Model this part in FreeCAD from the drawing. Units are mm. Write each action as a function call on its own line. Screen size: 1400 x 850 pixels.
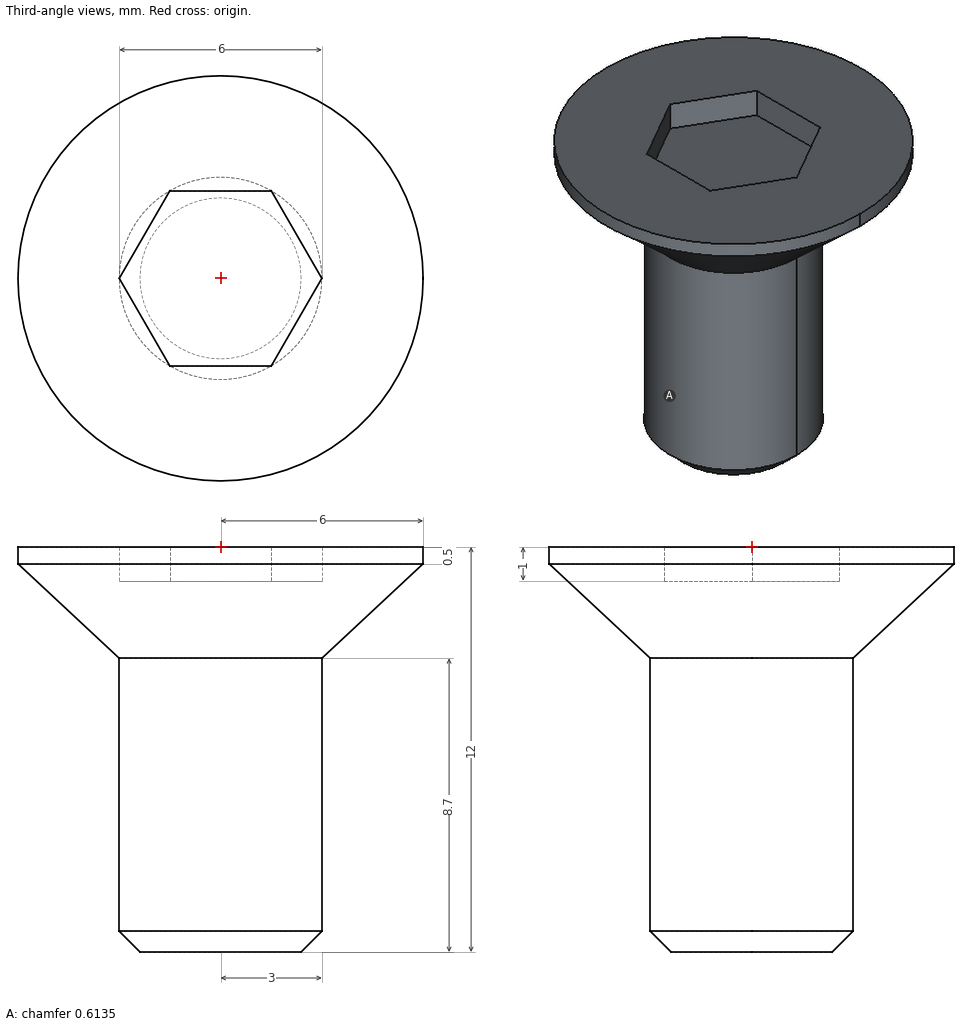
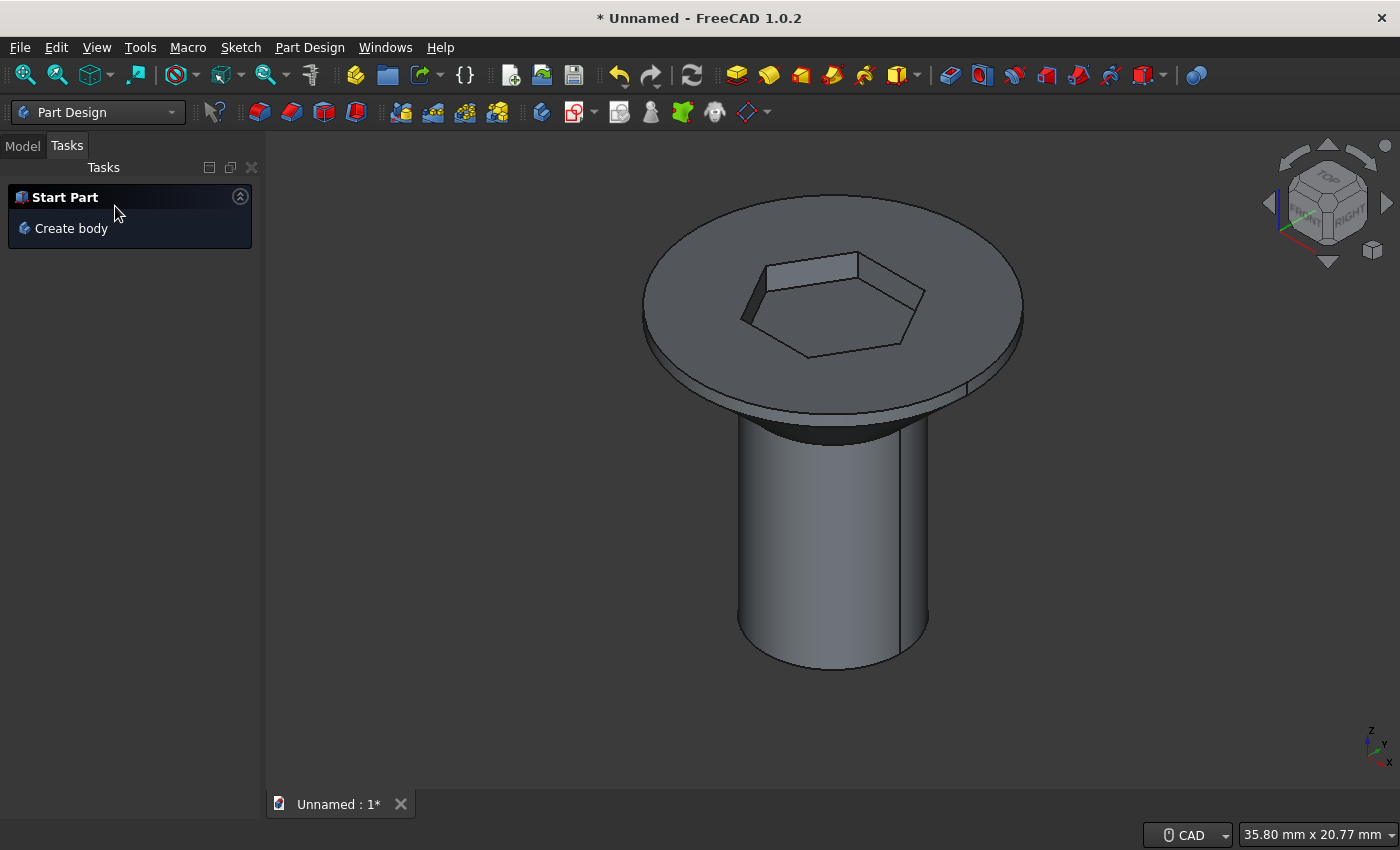
key(2)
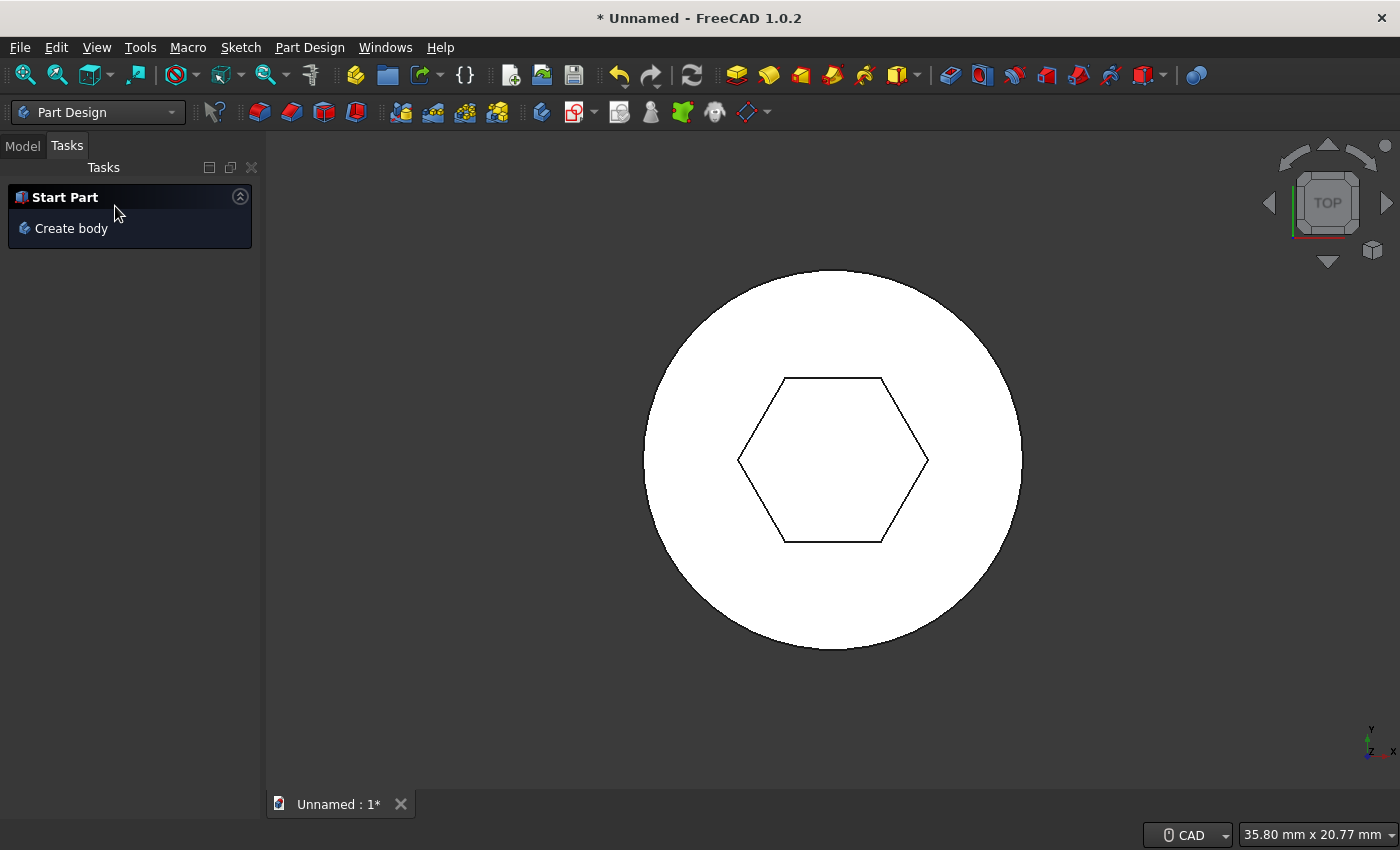
key(1)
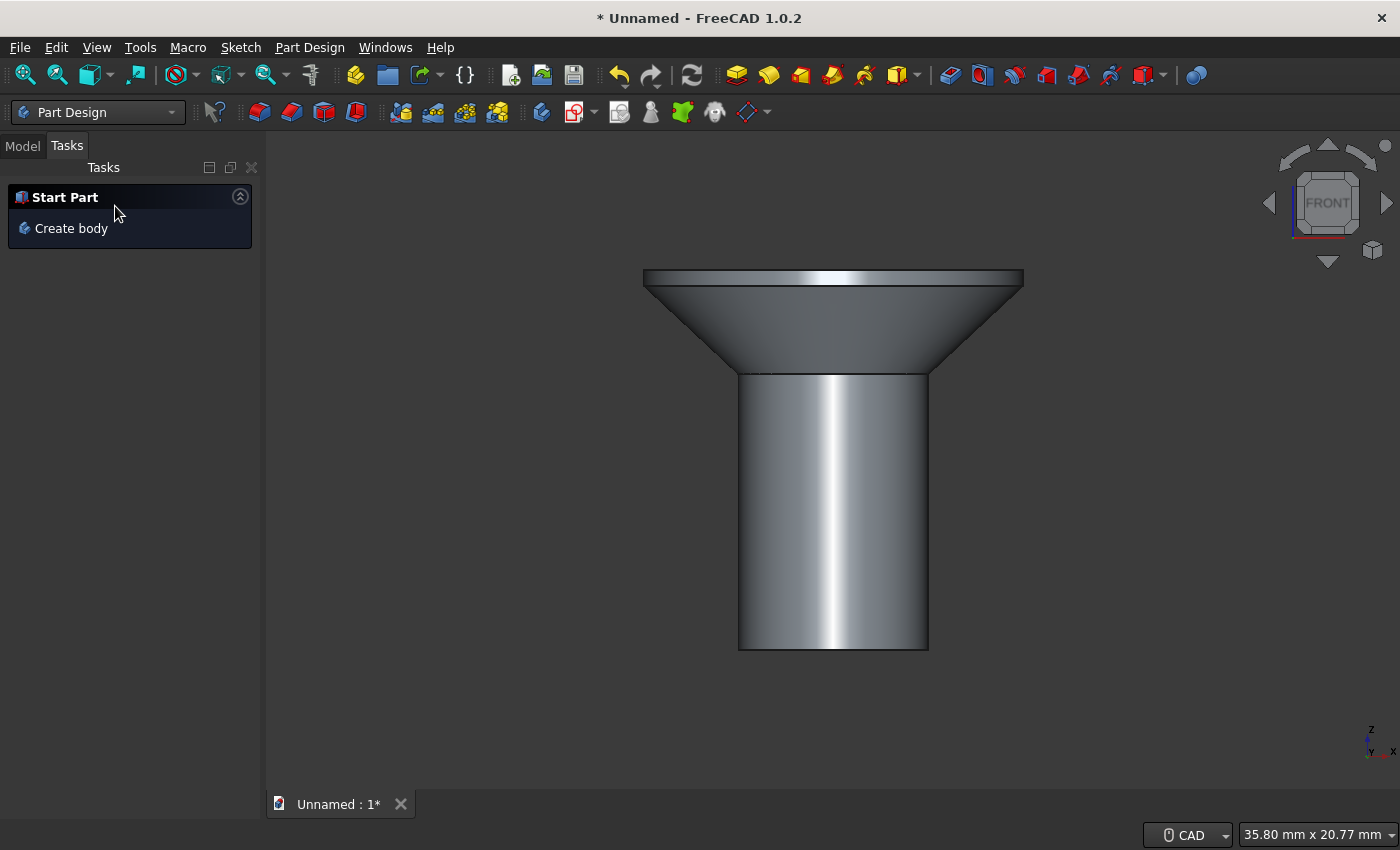
key(3)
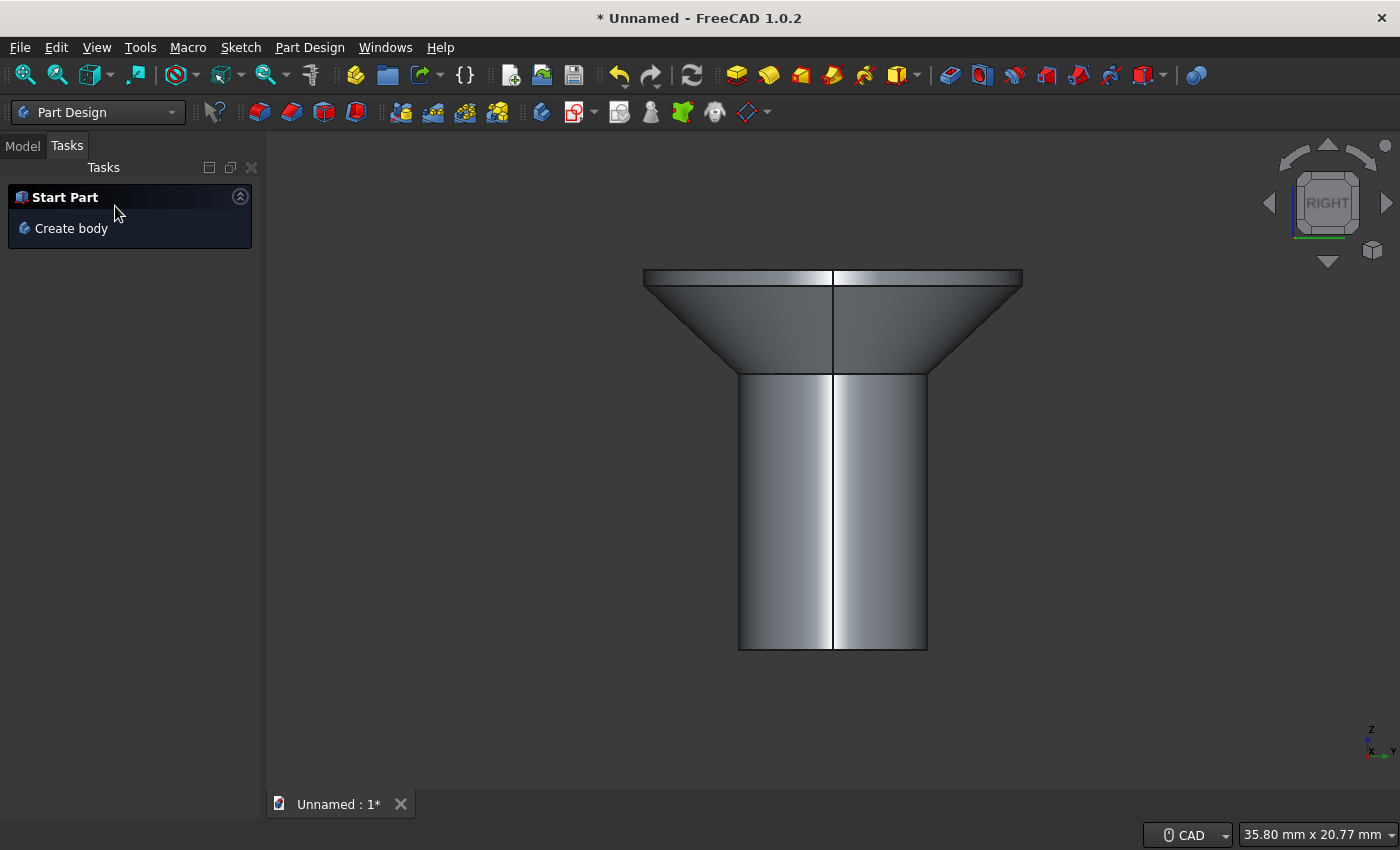
click(777, 649)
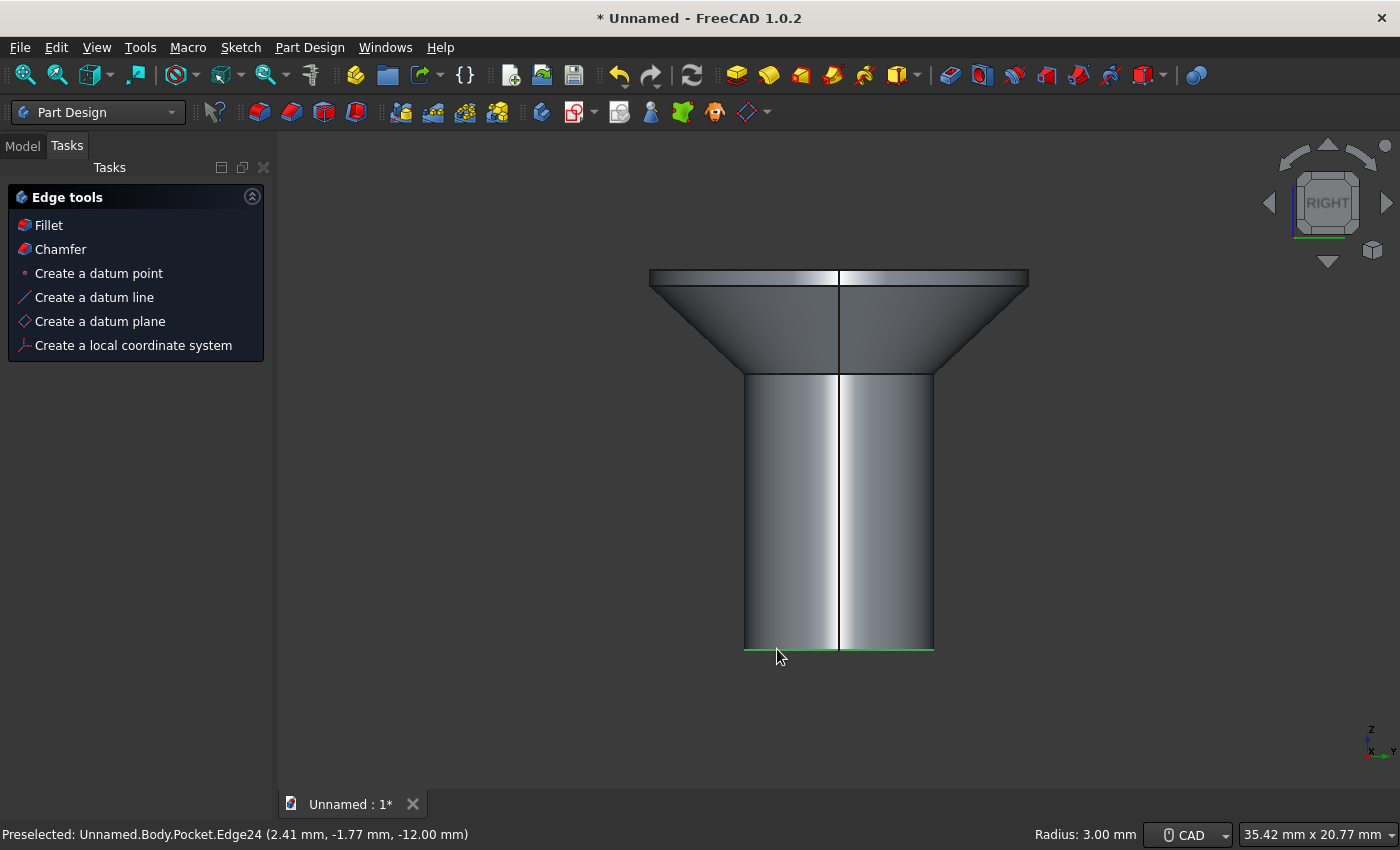
click(292, 112)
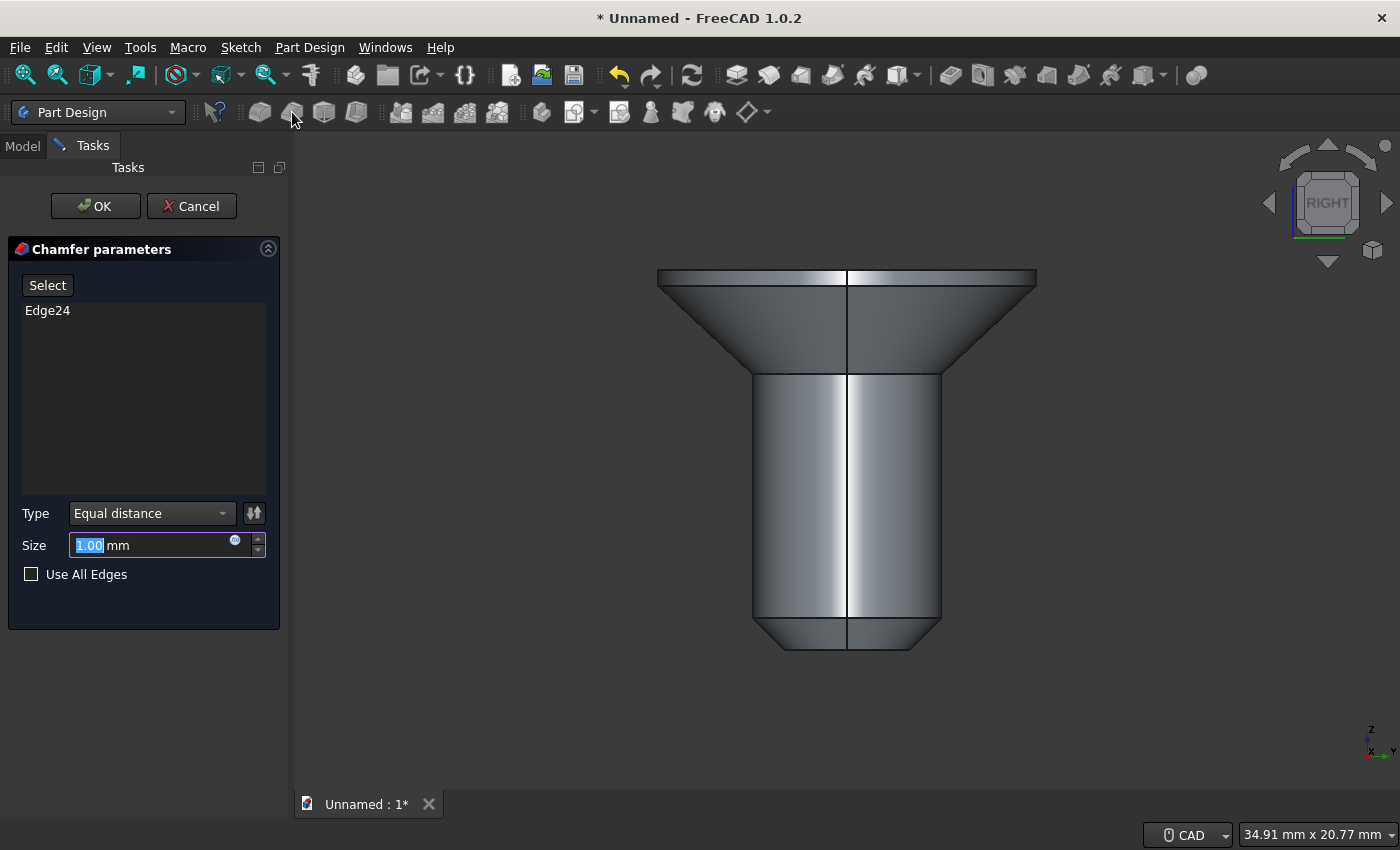
text(0.6135)
key(Tab)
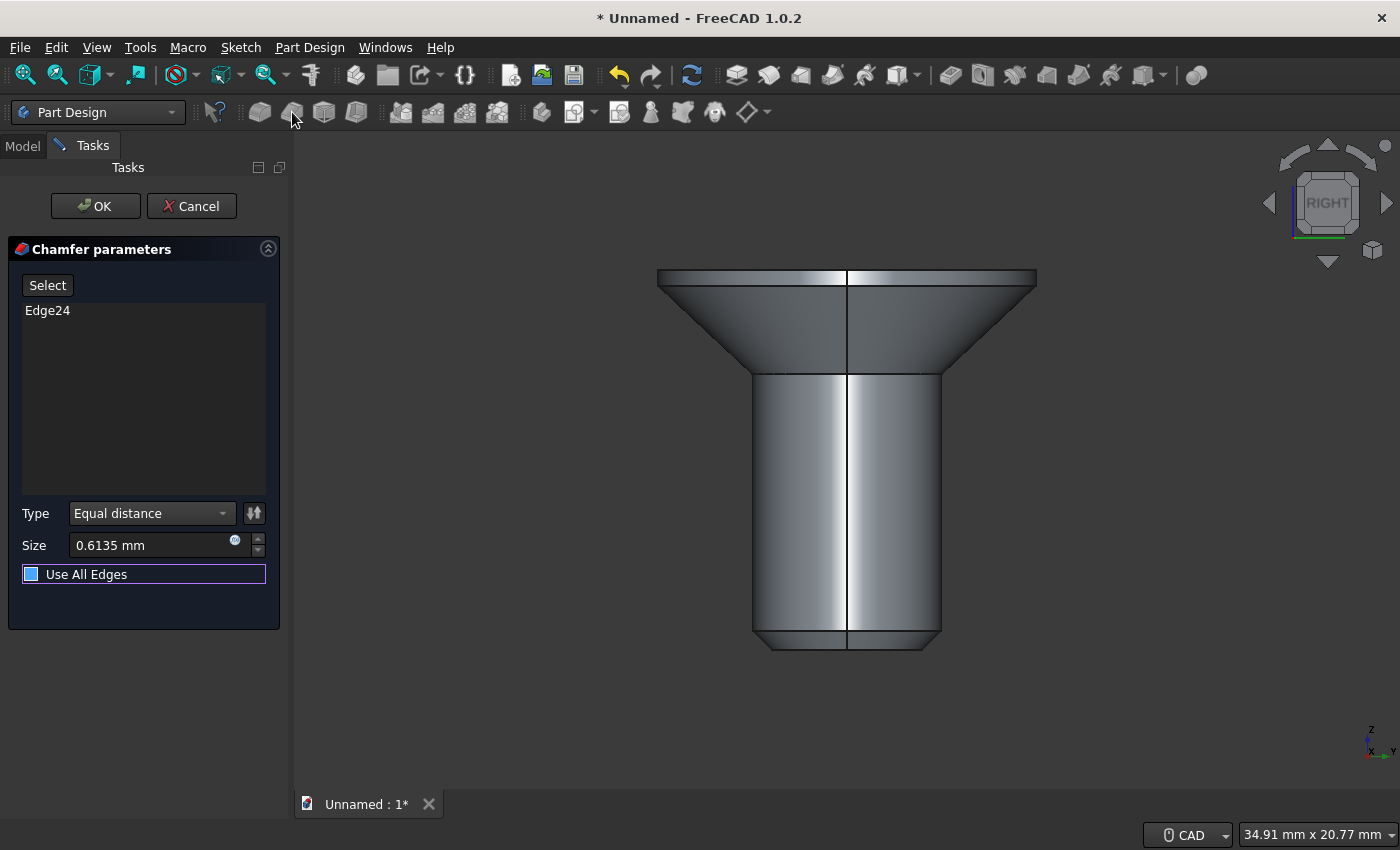
click(96, 206)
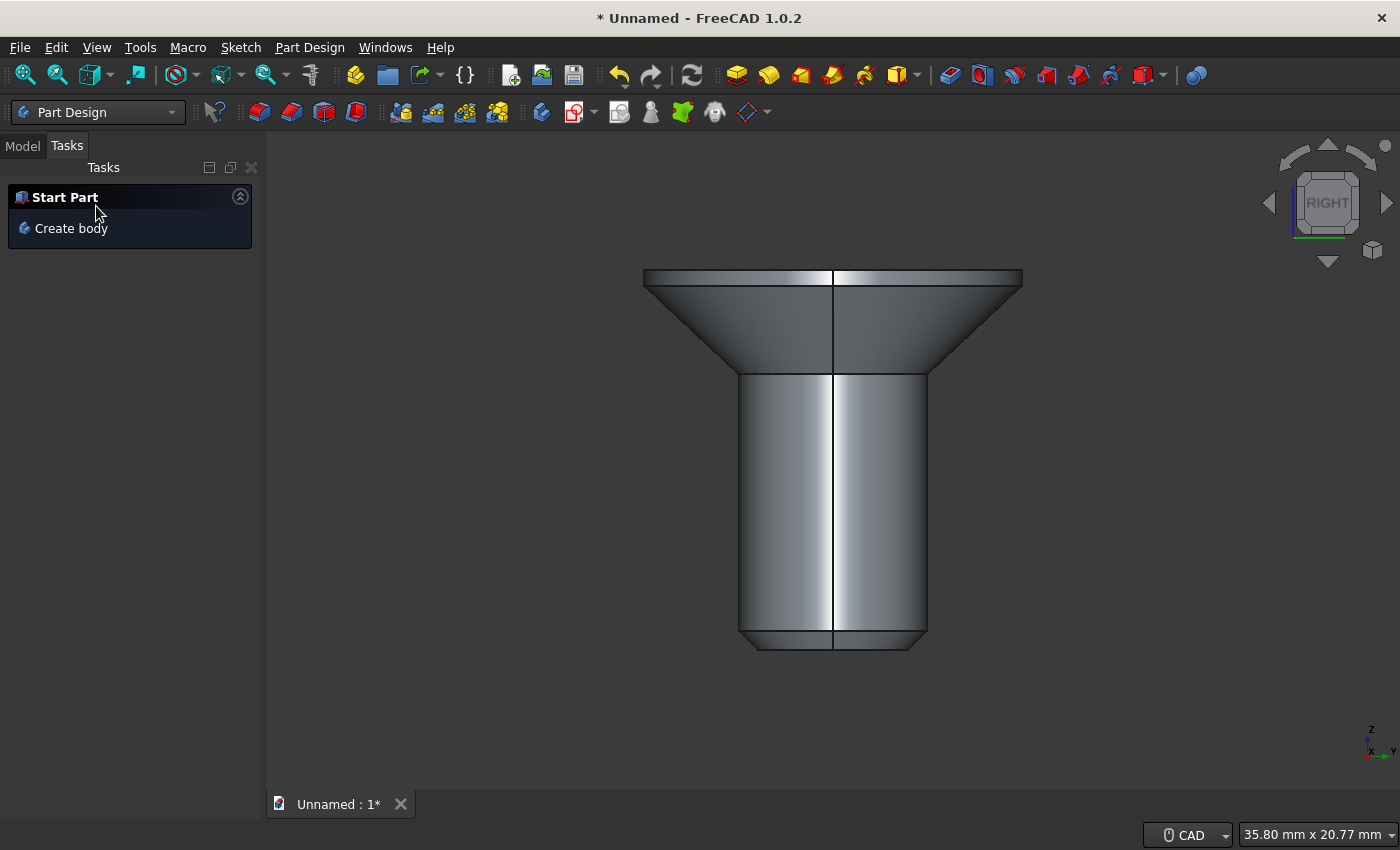
key(0)